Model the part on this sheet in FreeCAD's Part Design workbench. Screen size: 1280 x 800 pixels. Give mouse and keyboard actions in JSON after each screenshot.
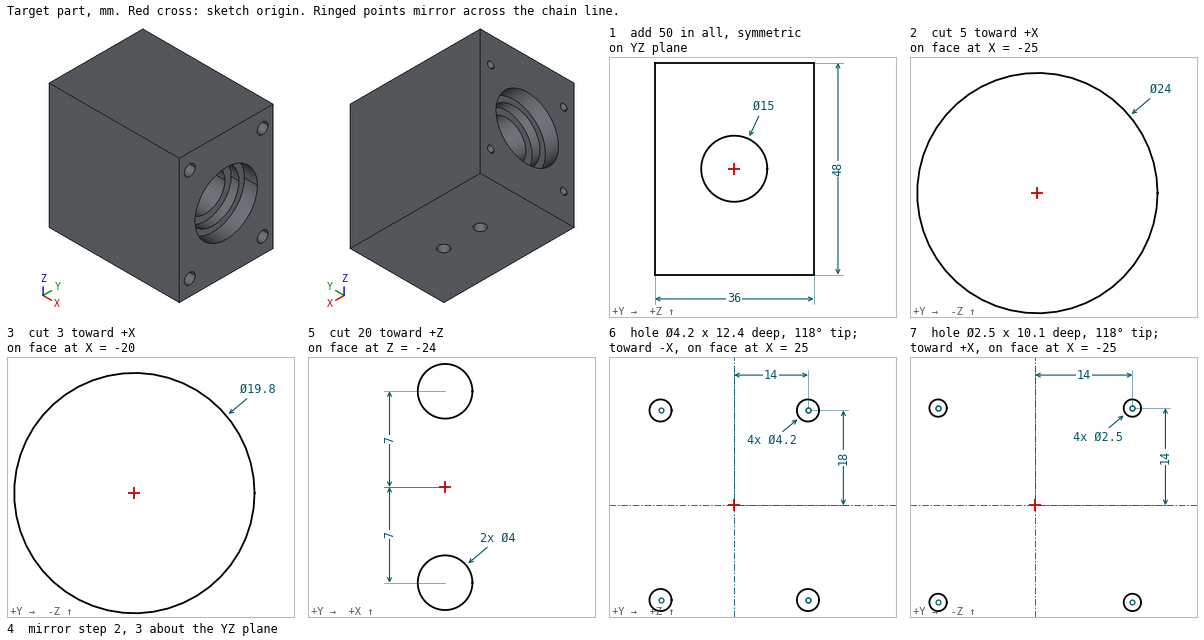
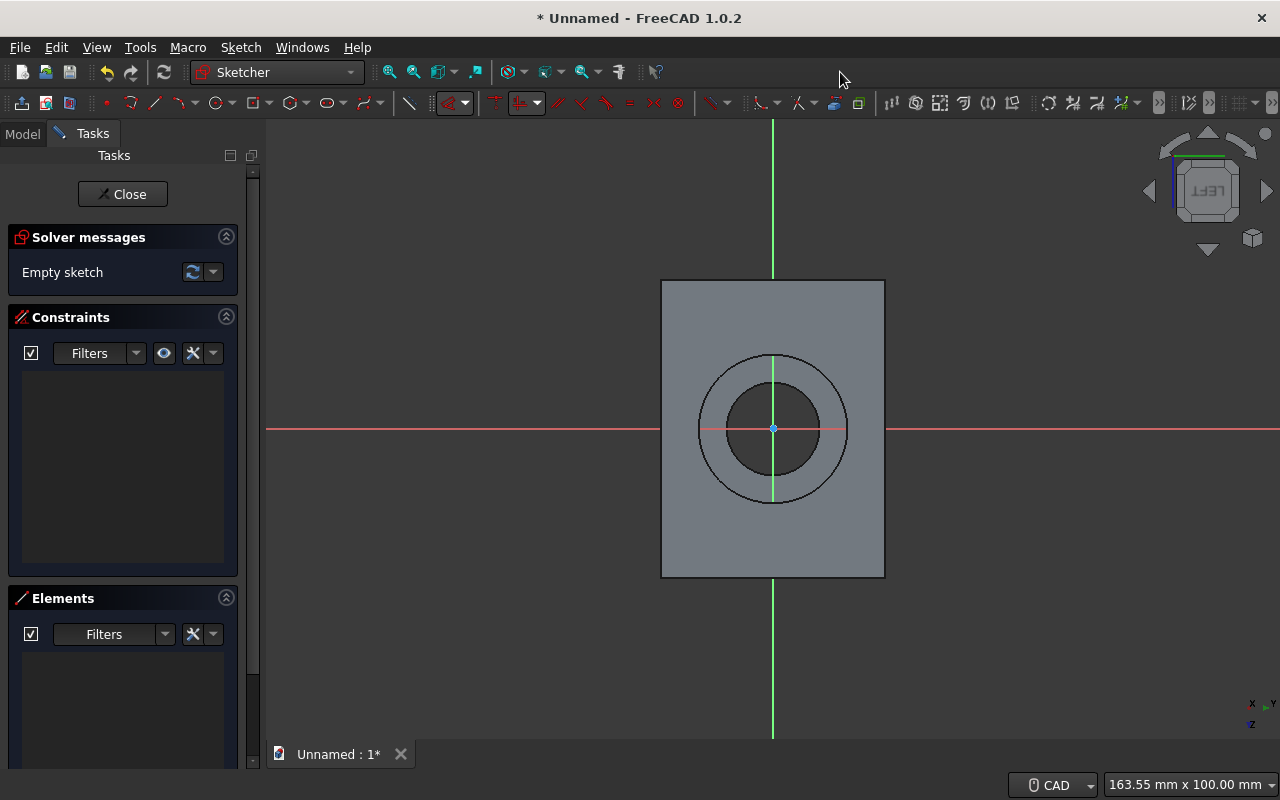
{"action": "left_click", "coordinate": [70, 104]}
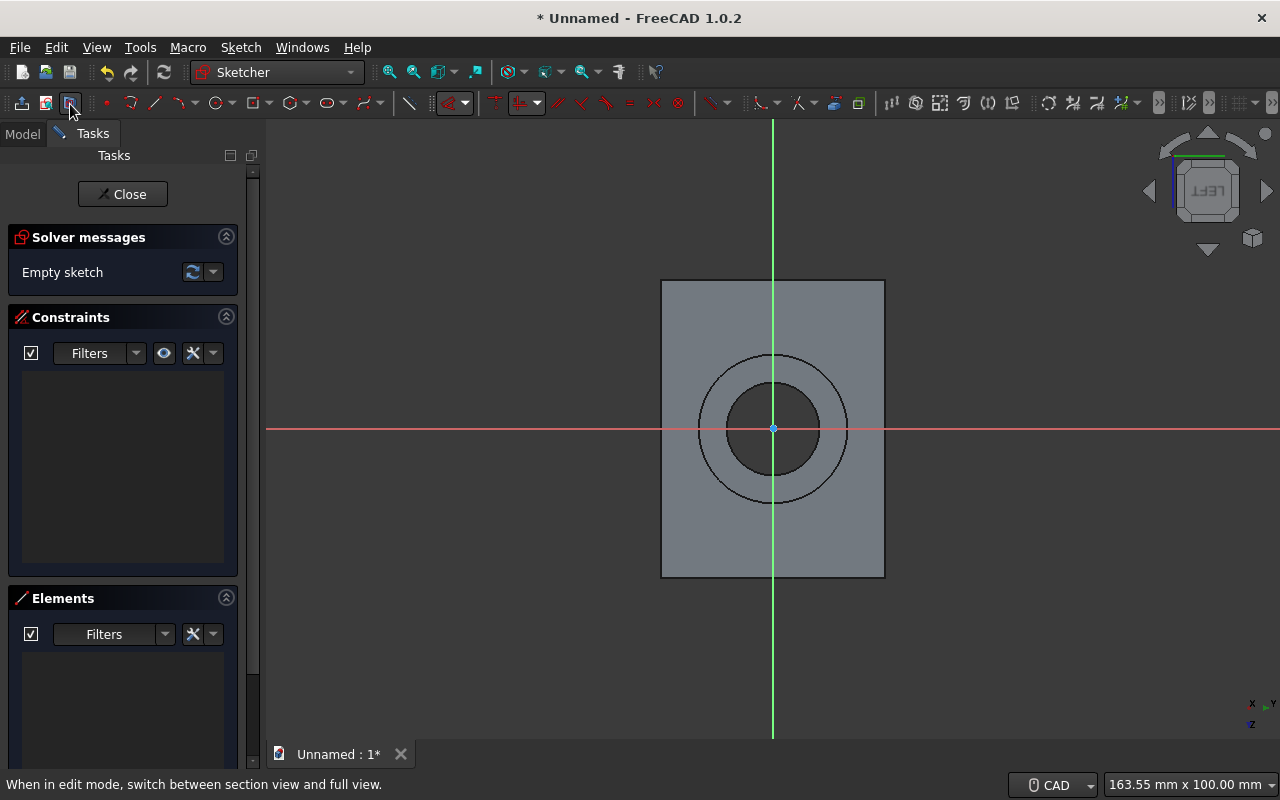
{"action": "scroll", "coordinate": [803, 429], "scroll_direction": "up", "scroll_amount": 6}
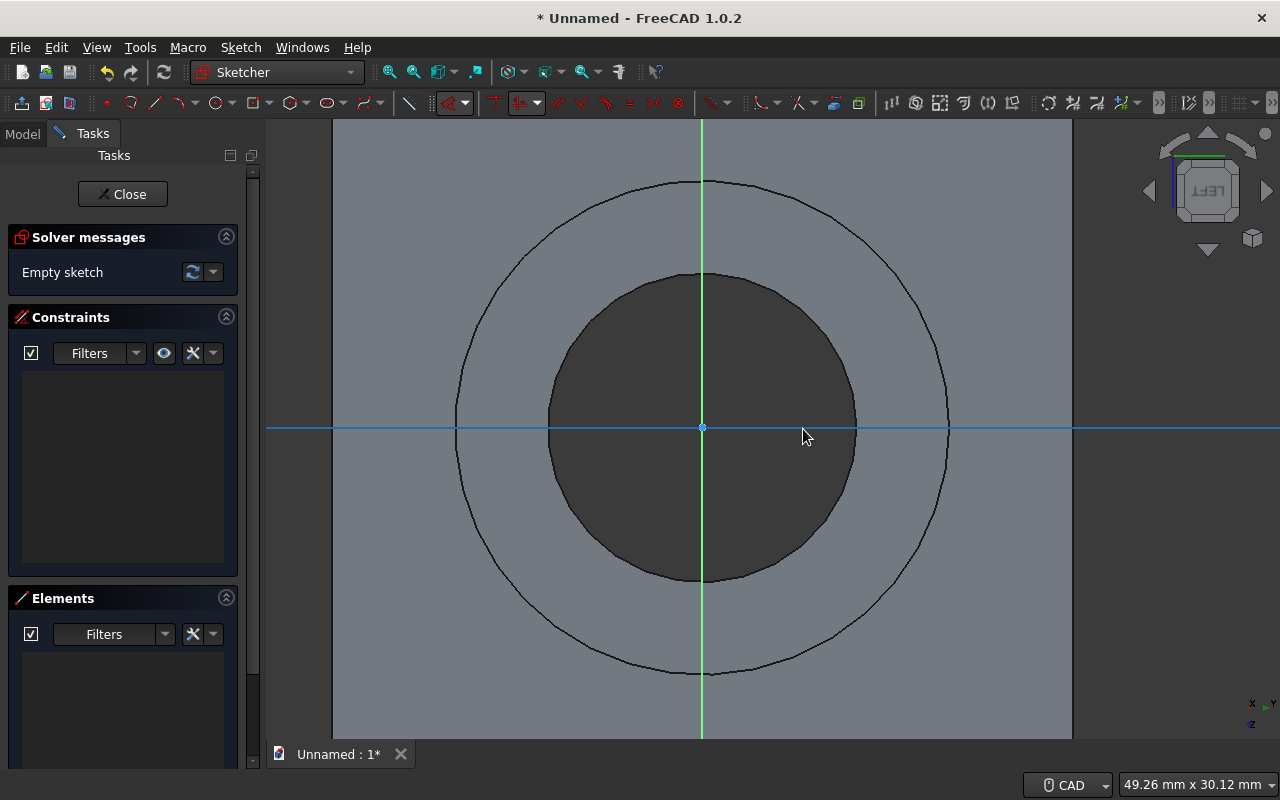
{"action": "left_click", "coordinate": [216, 104]}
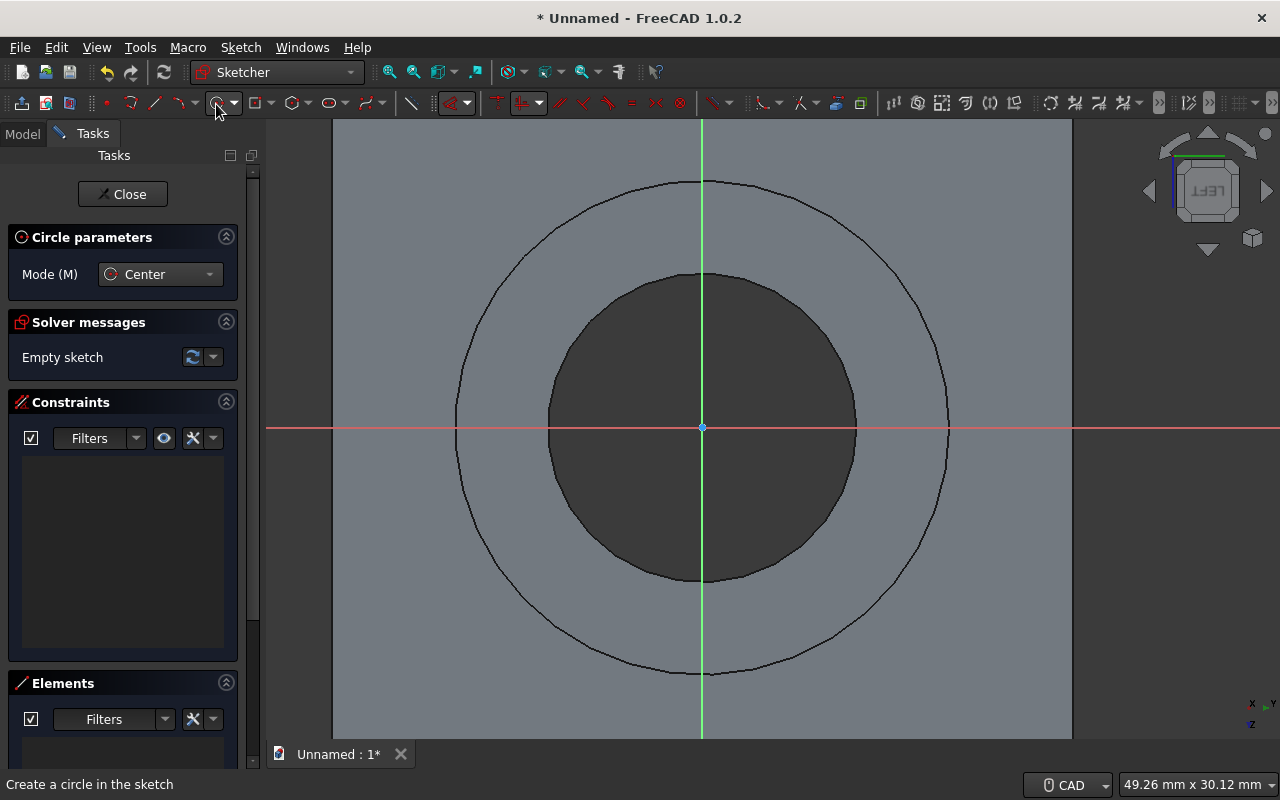
{"action": "left_click", "coordinate": [702, 428]}
{"action": "left_click", "coordinate": [846, 284]}
{"action": "key", "text": "Escape"}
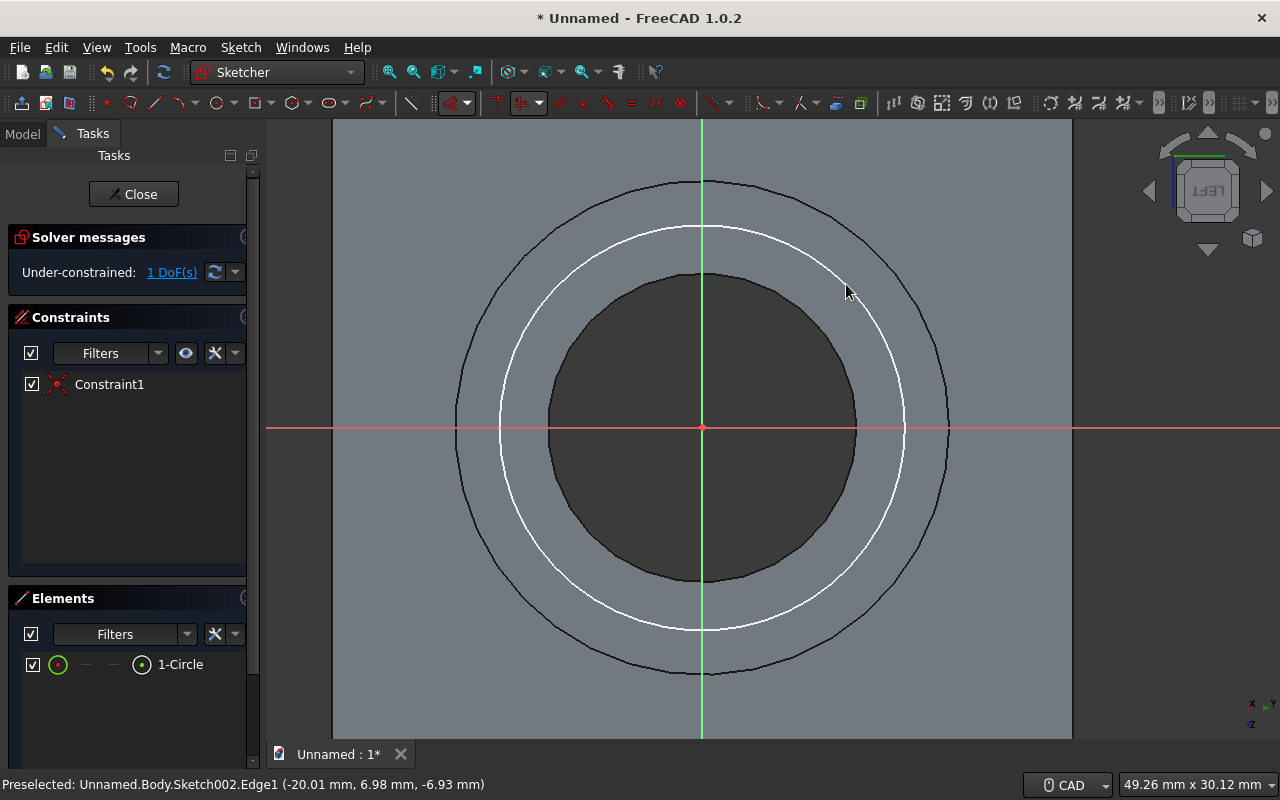
{"action": "left_click", "coordinate": [845, 284]}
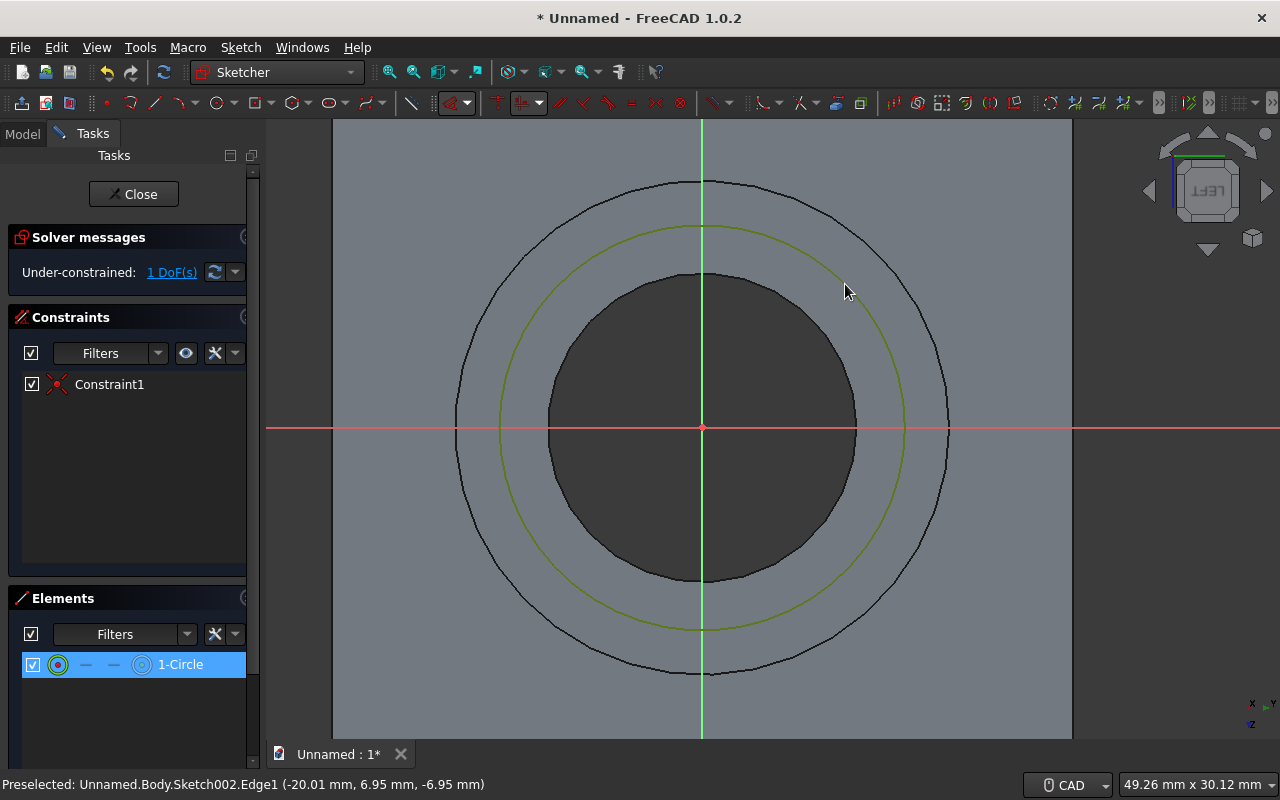
{"action": "left_click", "coordinate": [470, 104]}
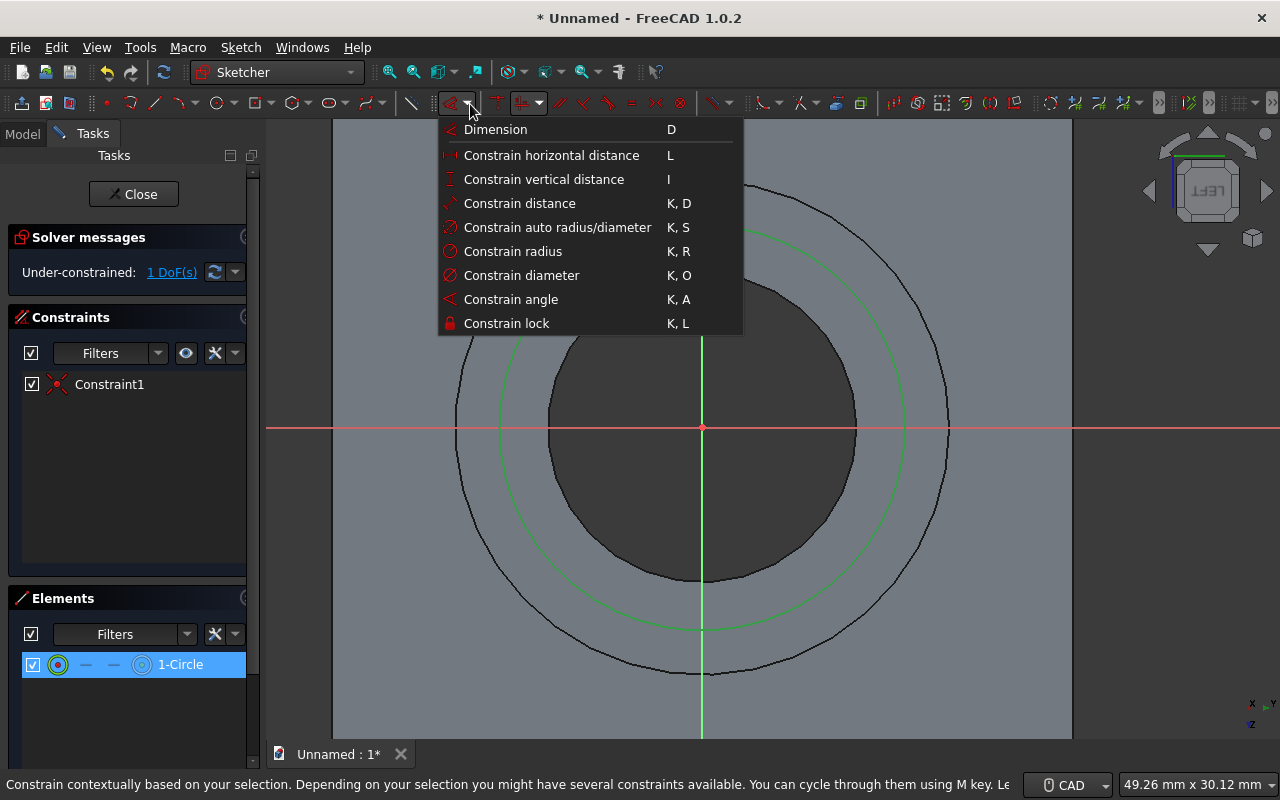
{"action": "left_click", "coordinate": [591, 275]}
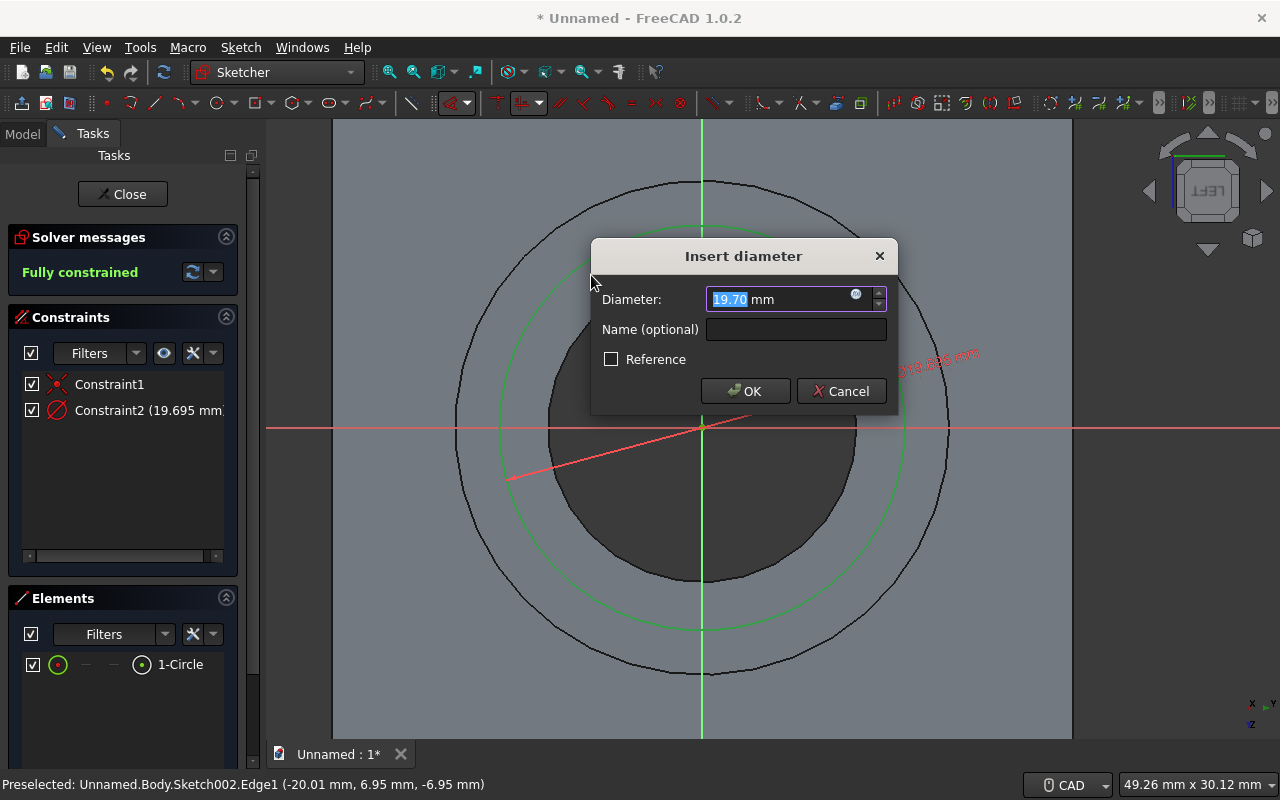
{"action": "type", "text": "19.8"}
{"action": "key", "text": "Return"}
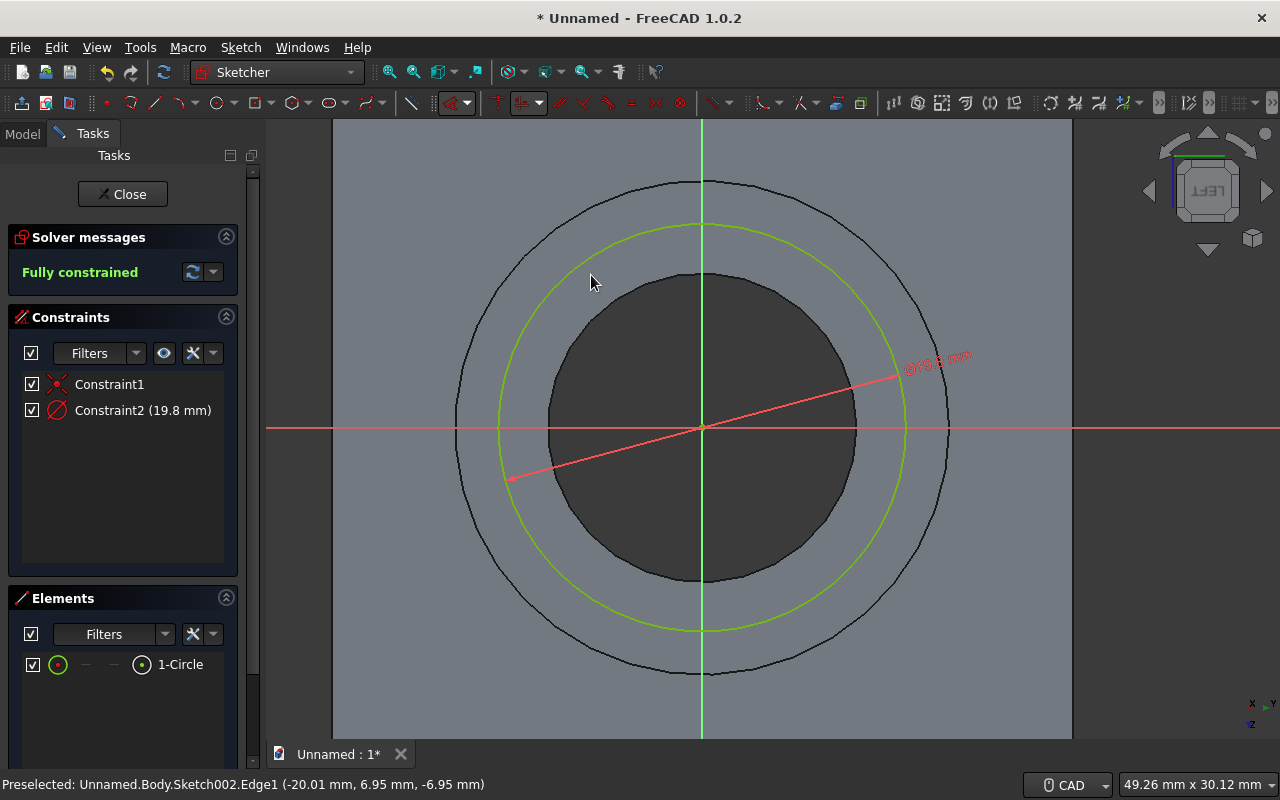
{"action": "left_click", "coordinate": [123, 194]}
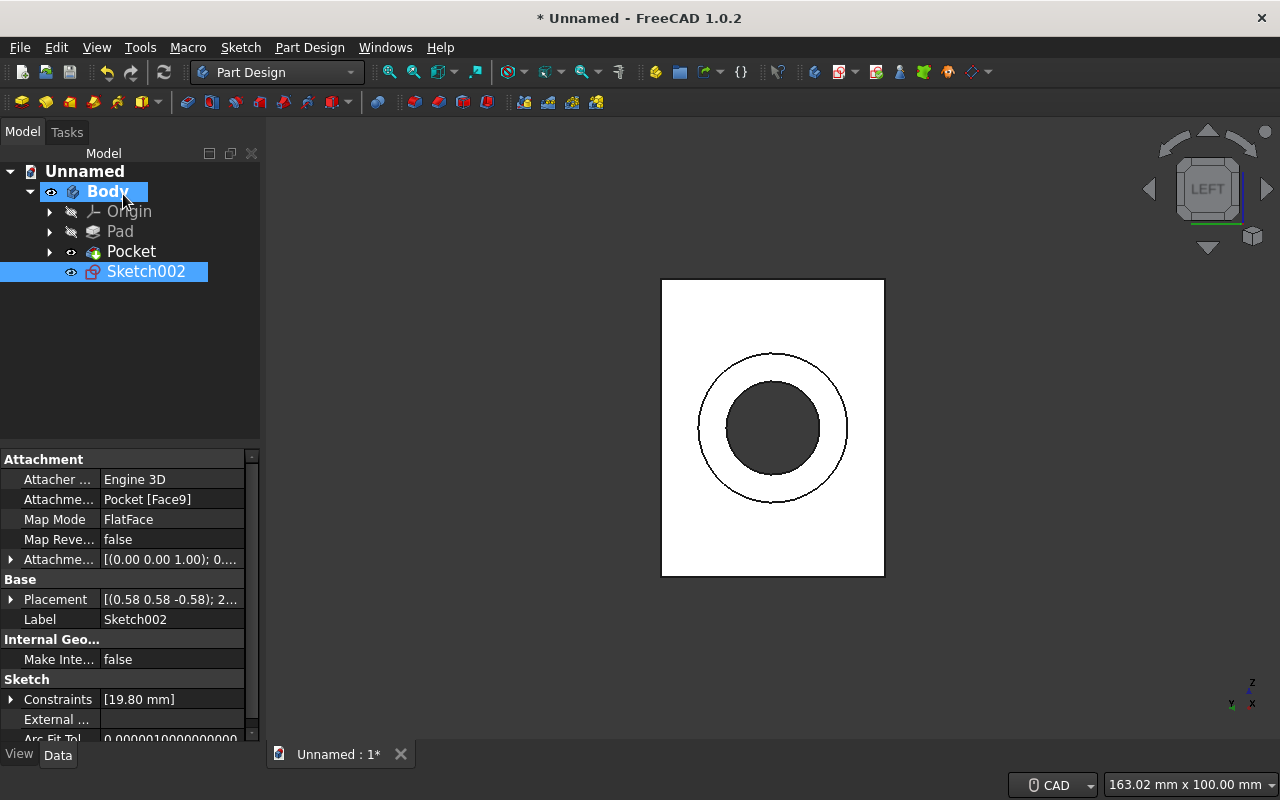
{"action": "left_click", "coordinate": [188, 102]}